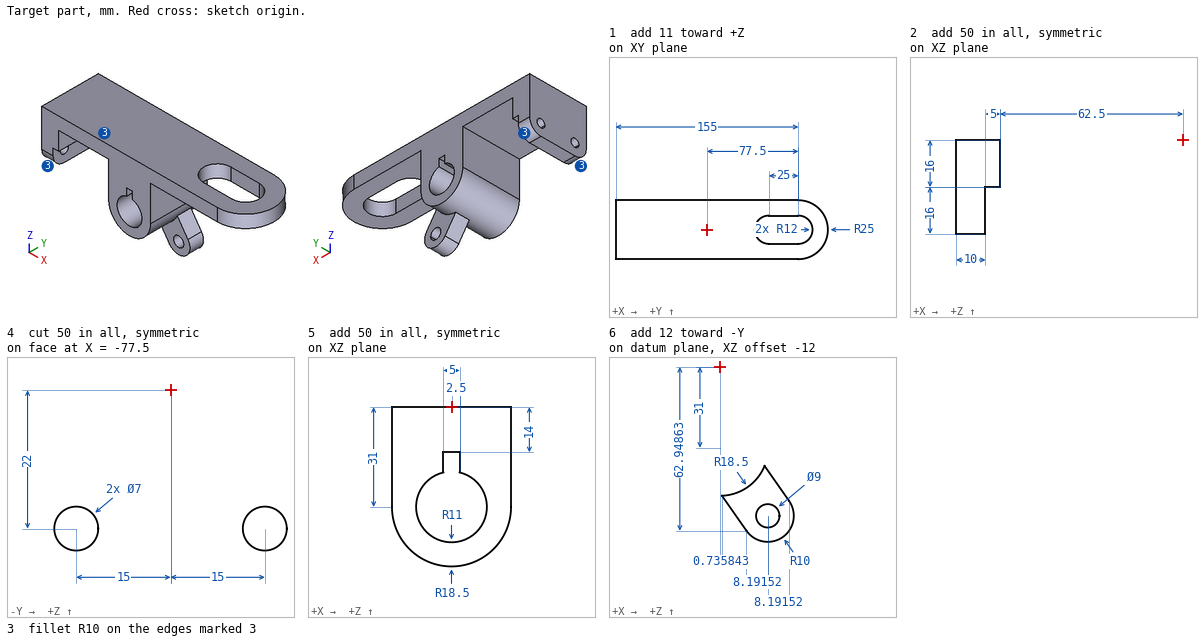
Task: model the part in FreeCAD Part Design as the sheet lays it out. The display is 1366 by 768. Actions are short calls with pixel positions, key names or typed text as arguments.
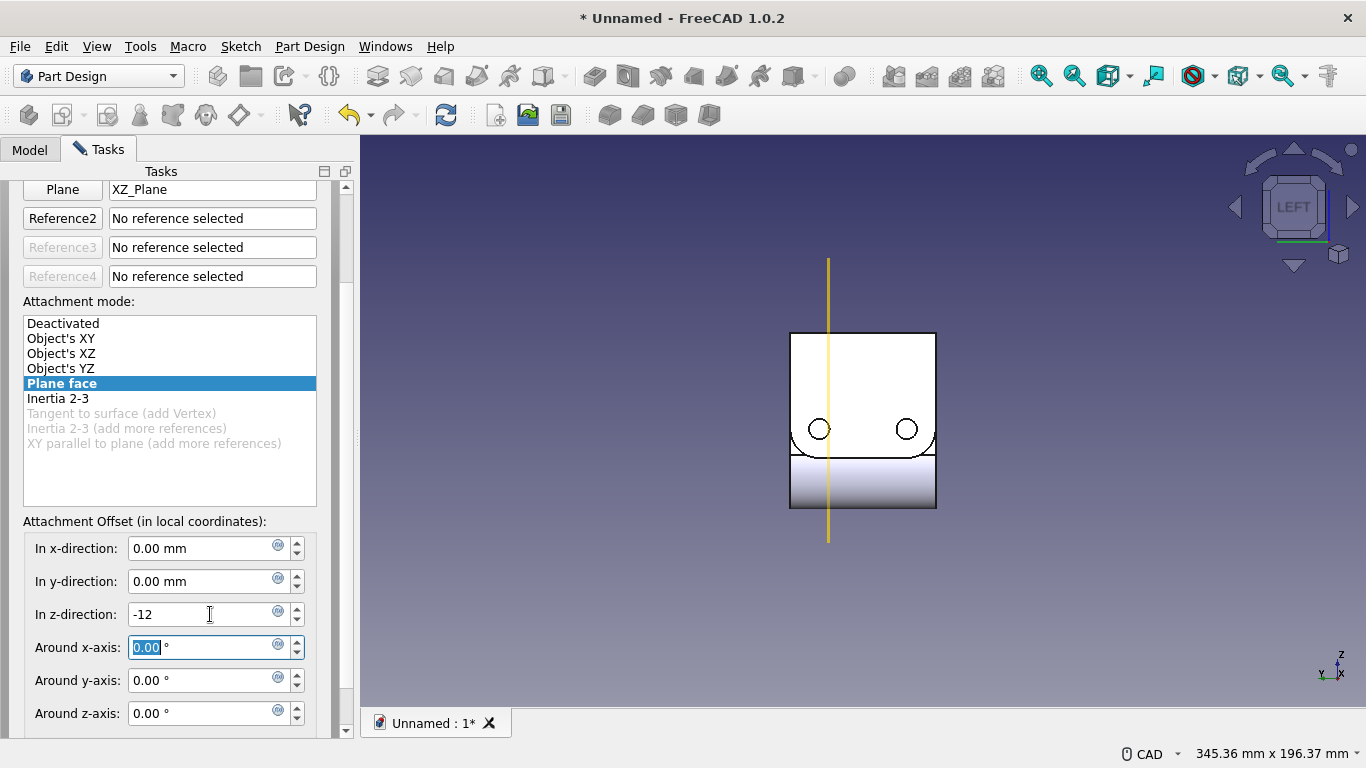
scroll(346, 460, up, 3)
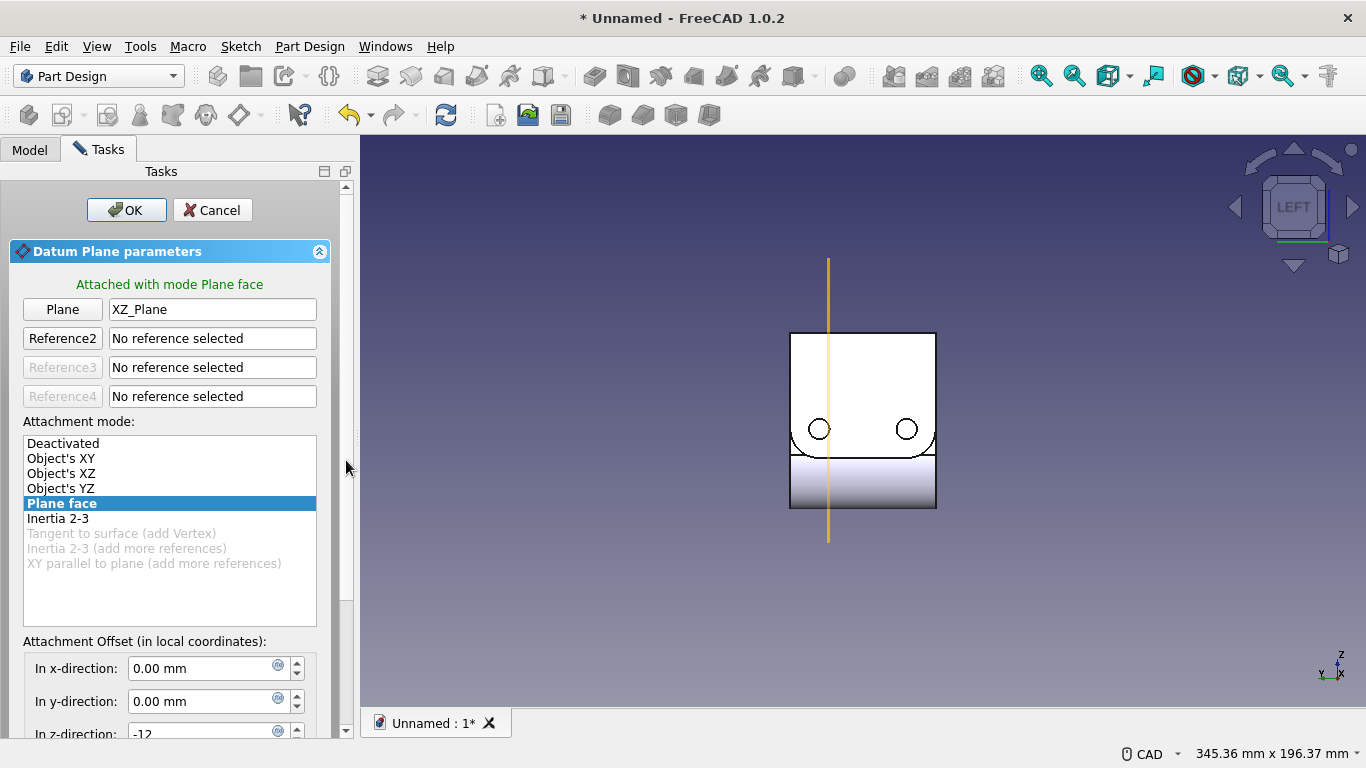
click(127, 210)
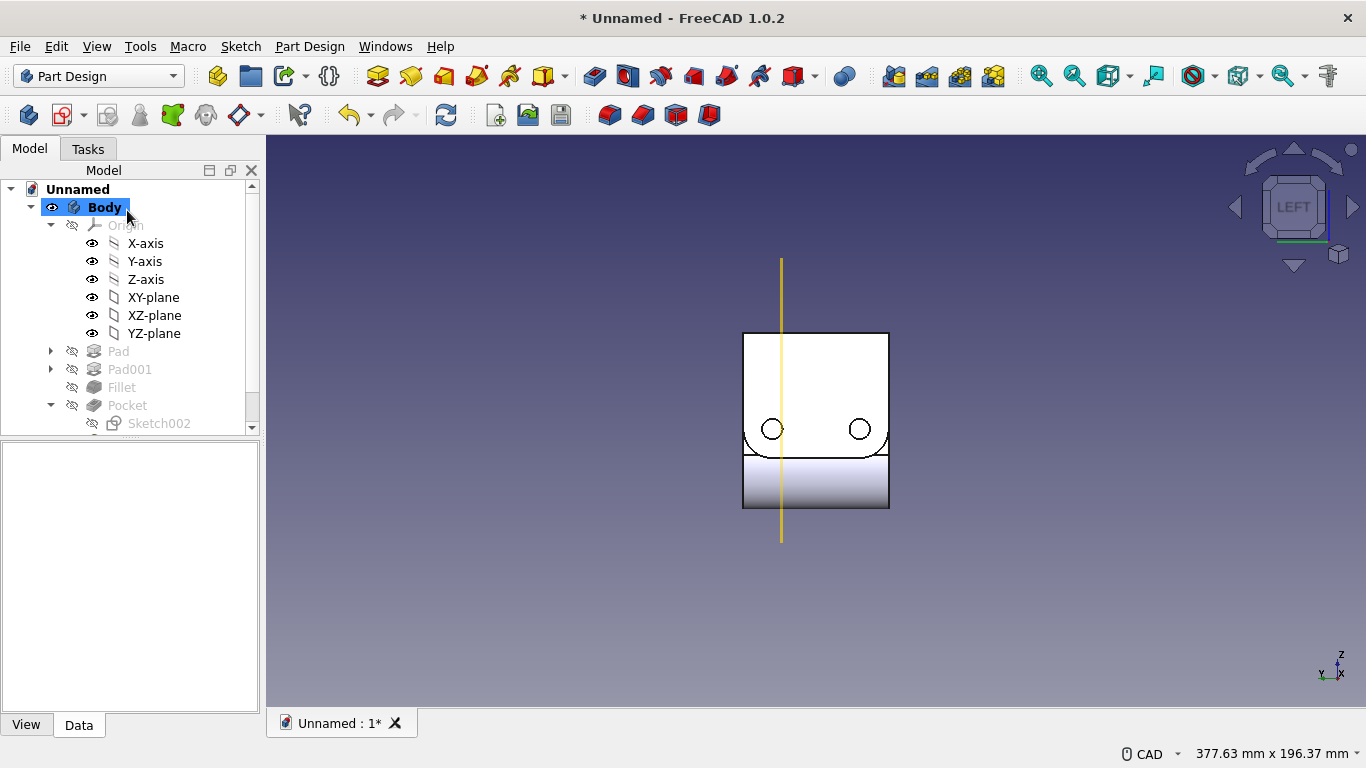
scroll(101, 311, down, 3)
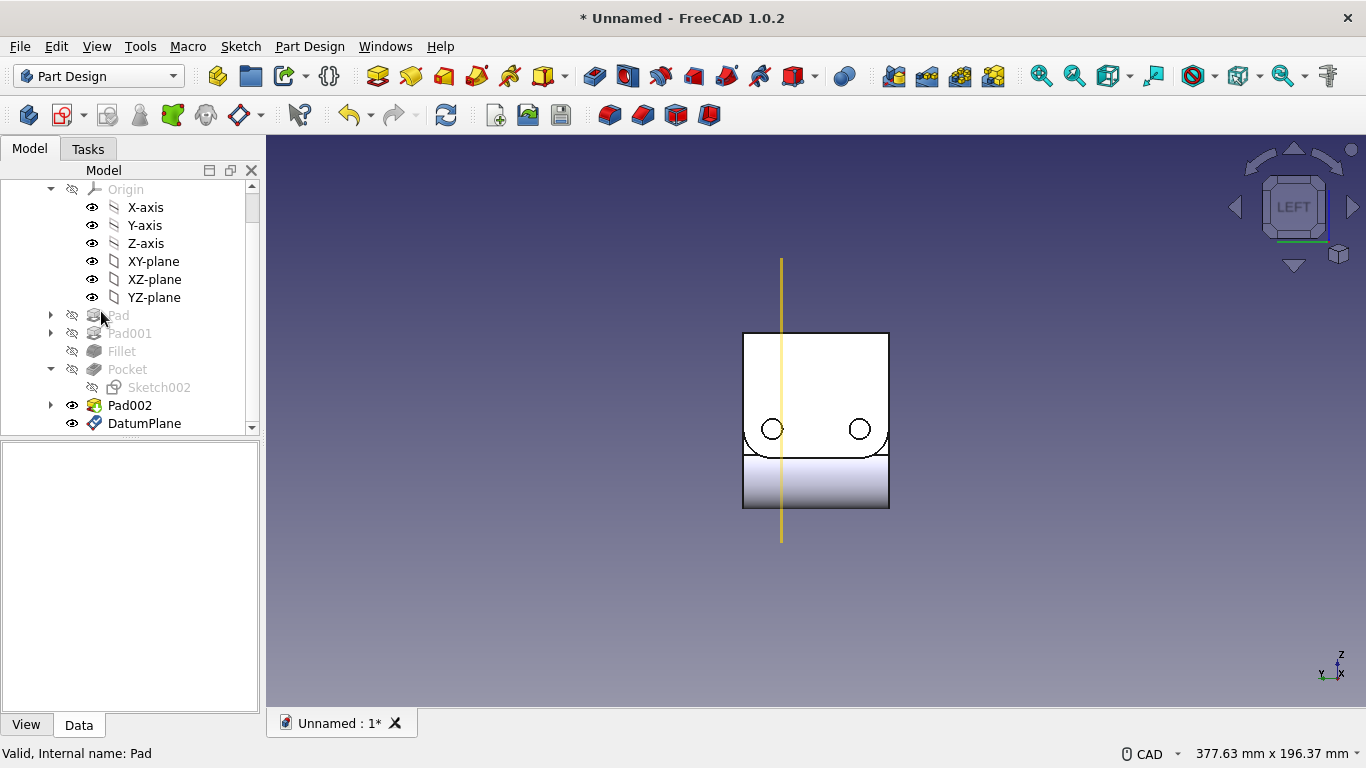
click(117, 423)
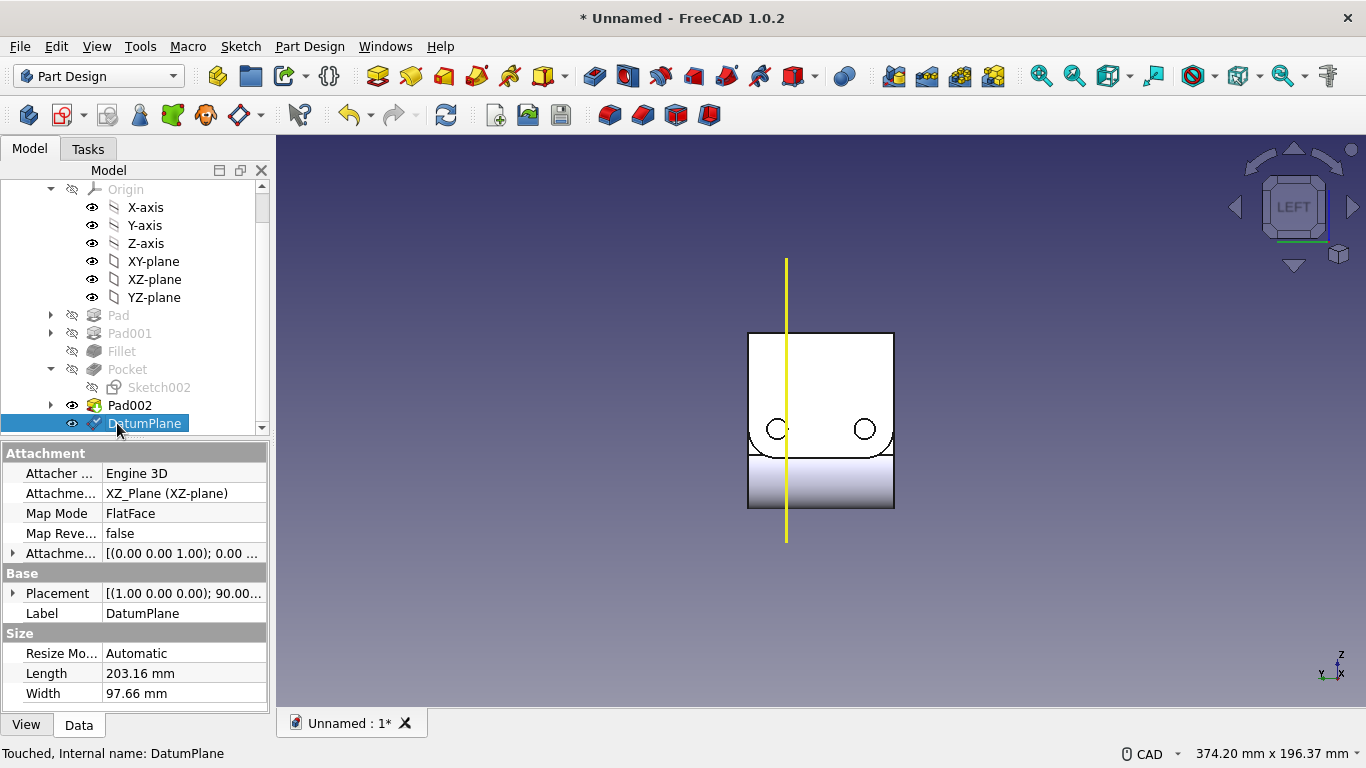
click(62, 116)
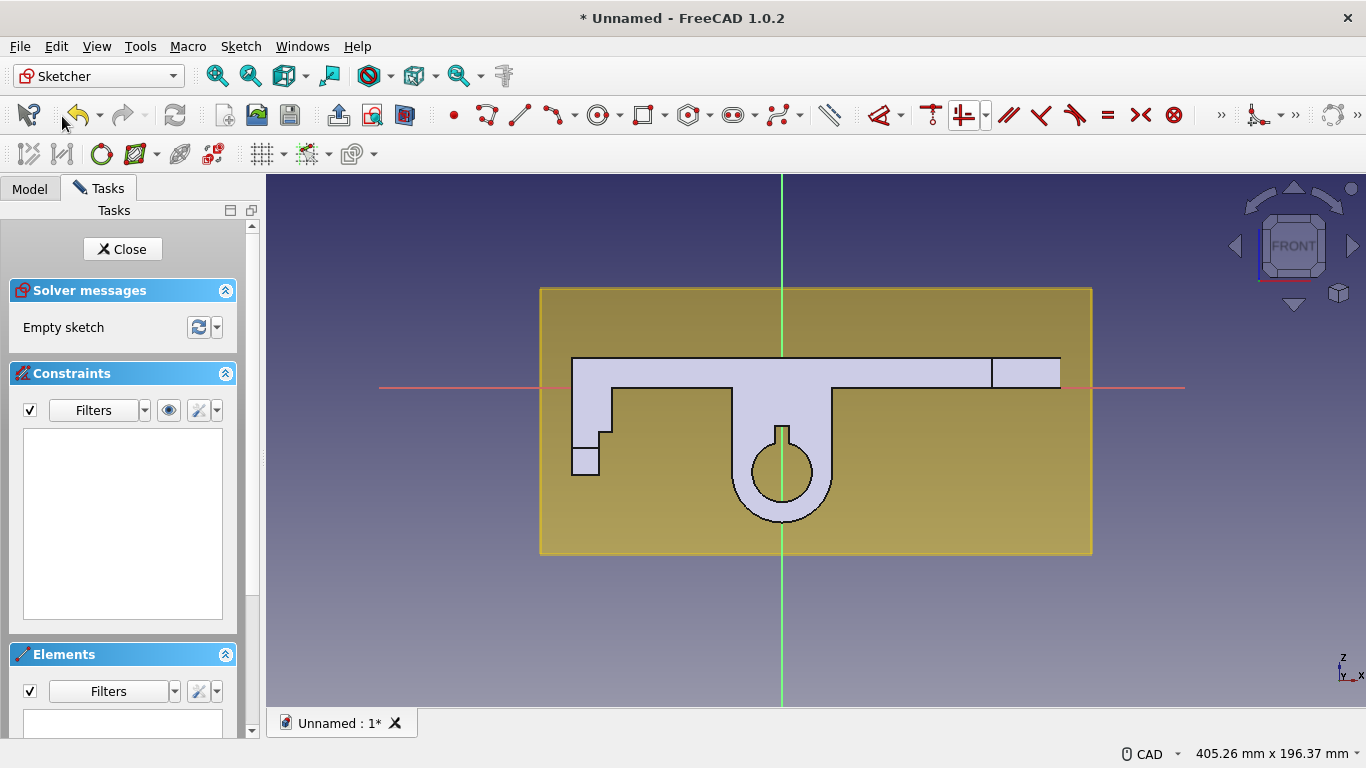
key(q)
key(s)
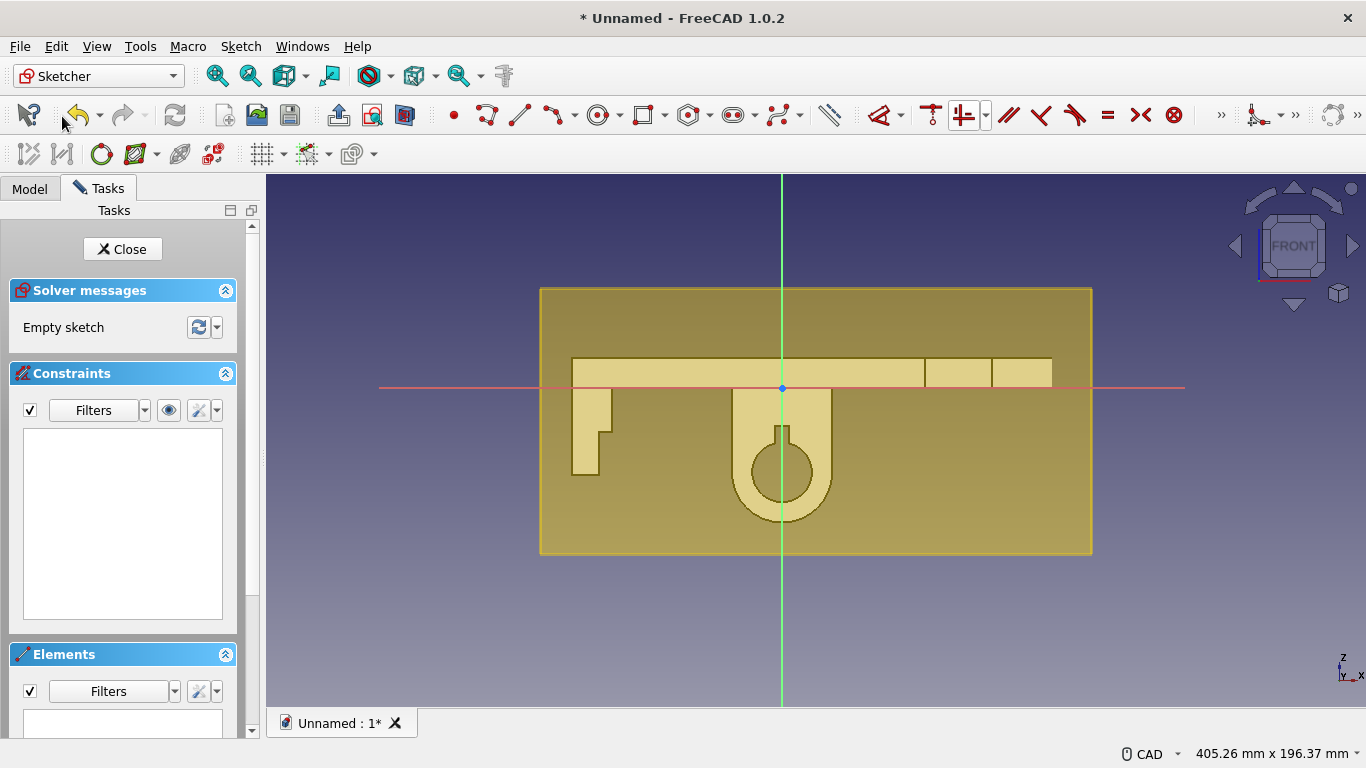
scroll(904, 521, up, 3)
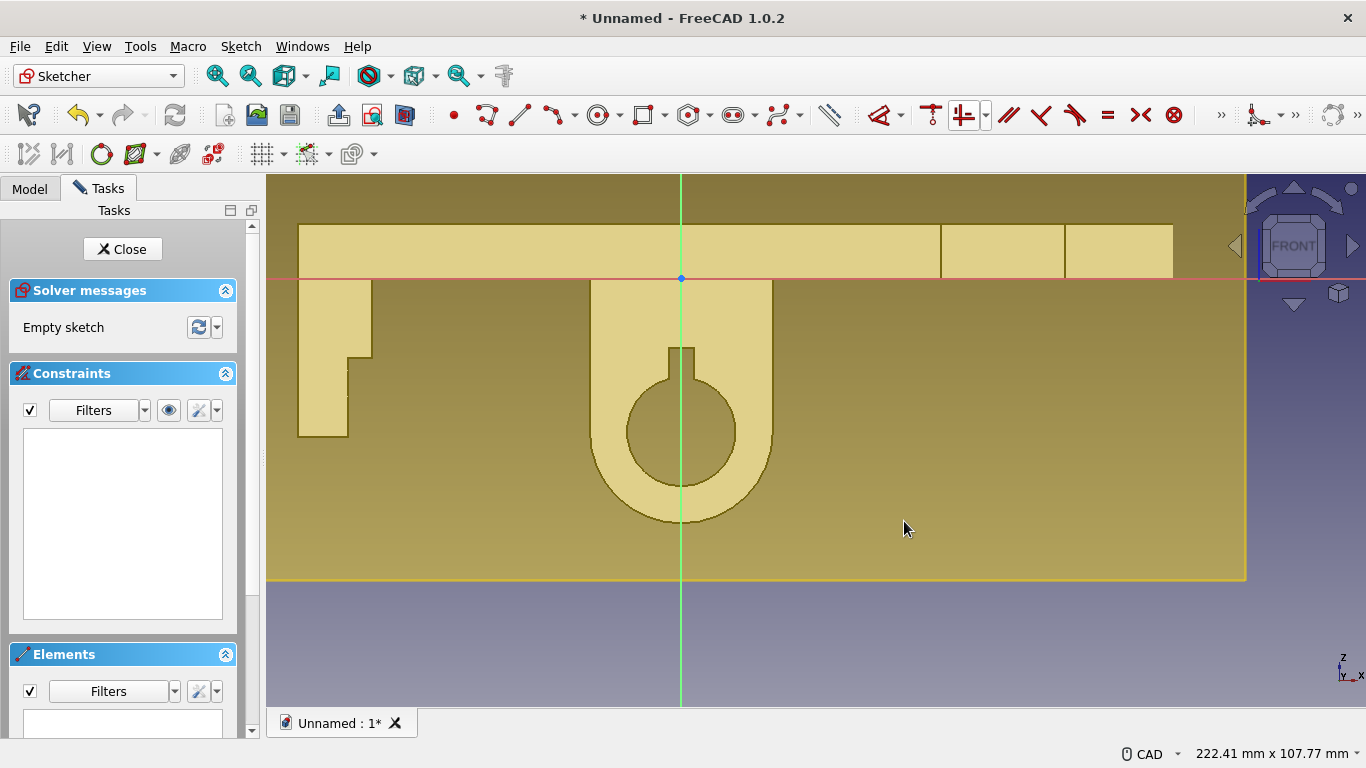
click(520, 116)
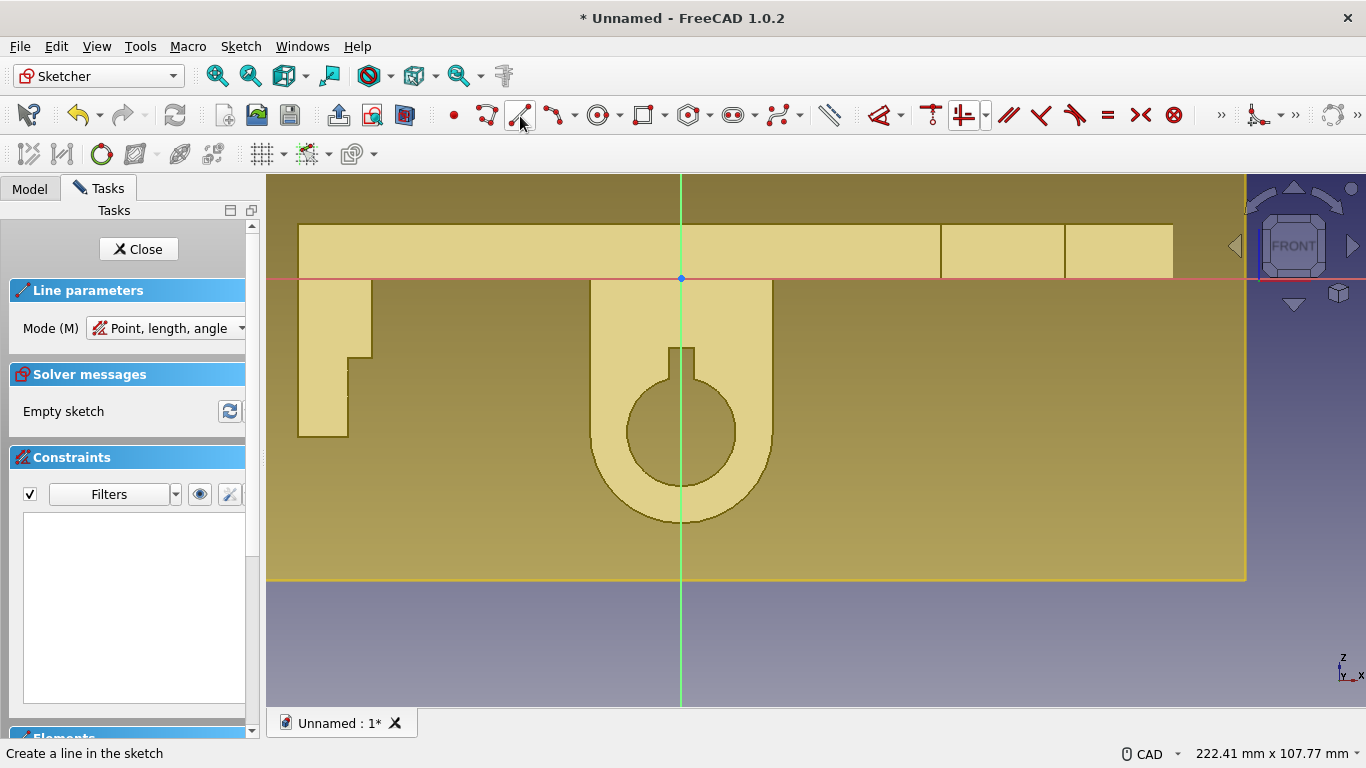
click(766, 467)
click(813, 533)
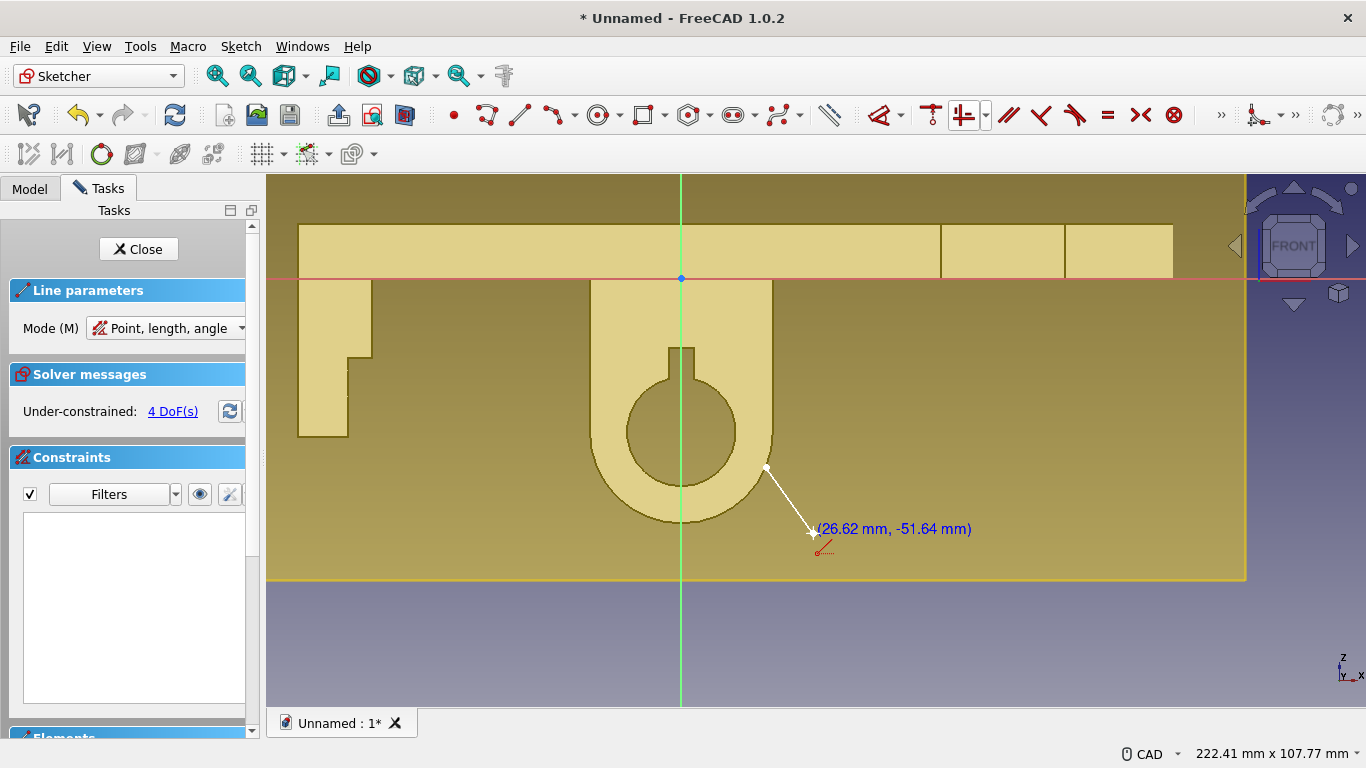
click(732, 590)